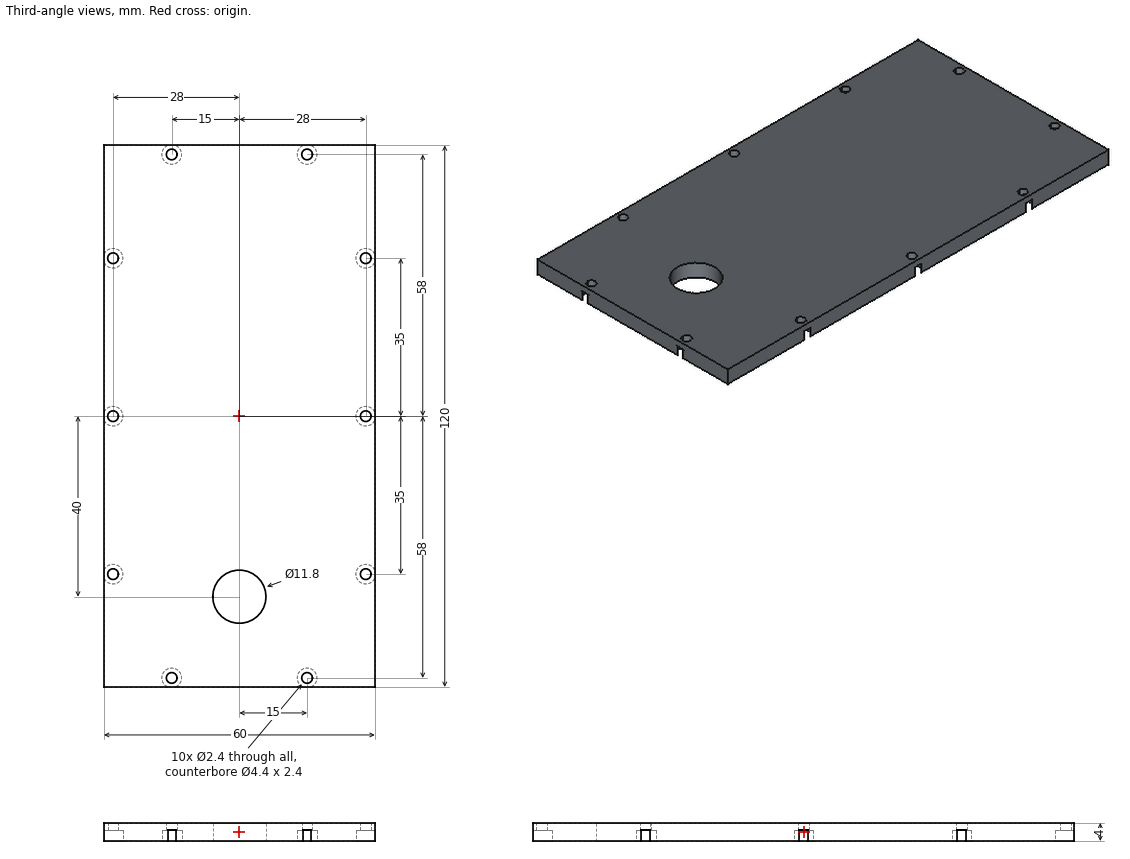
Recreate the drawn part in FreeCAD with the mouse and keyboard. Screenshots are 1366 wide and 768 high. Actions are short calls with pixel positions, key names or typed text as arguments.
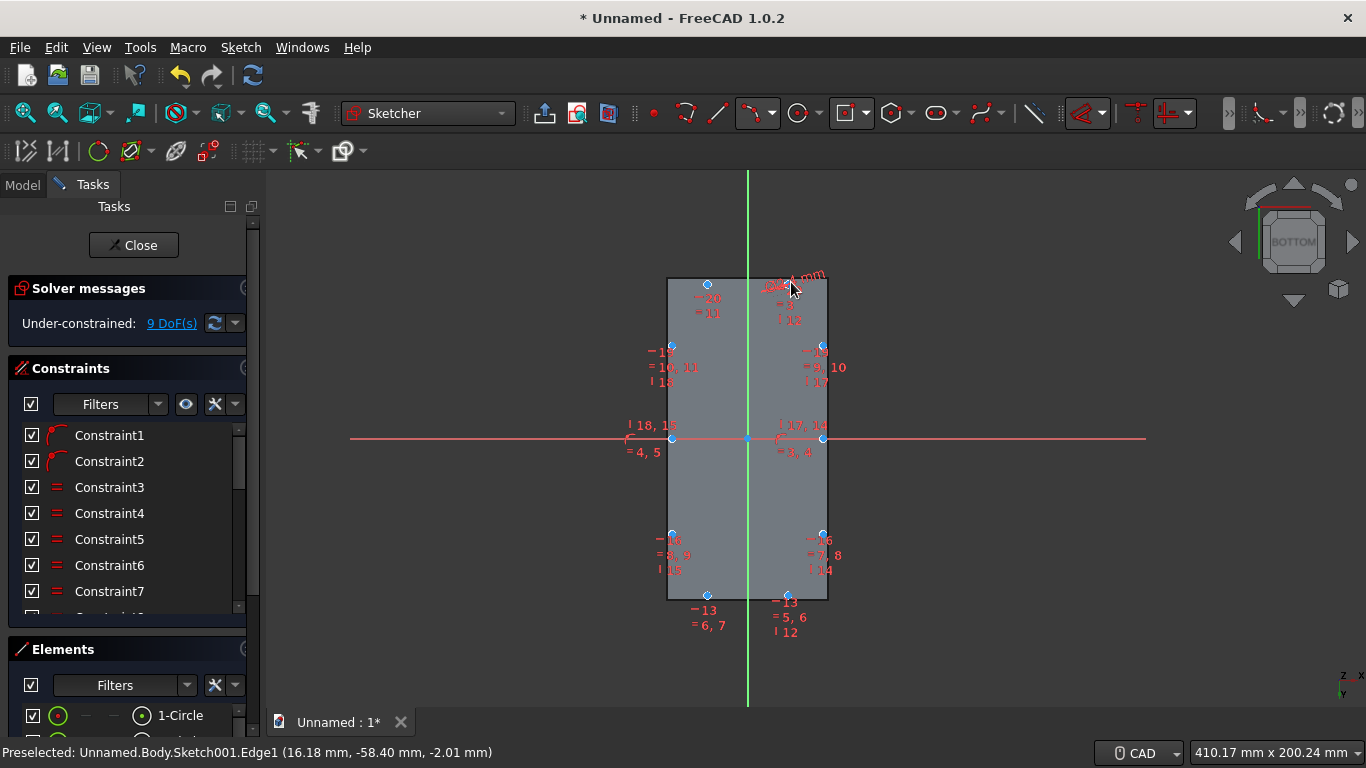
click(788, 284)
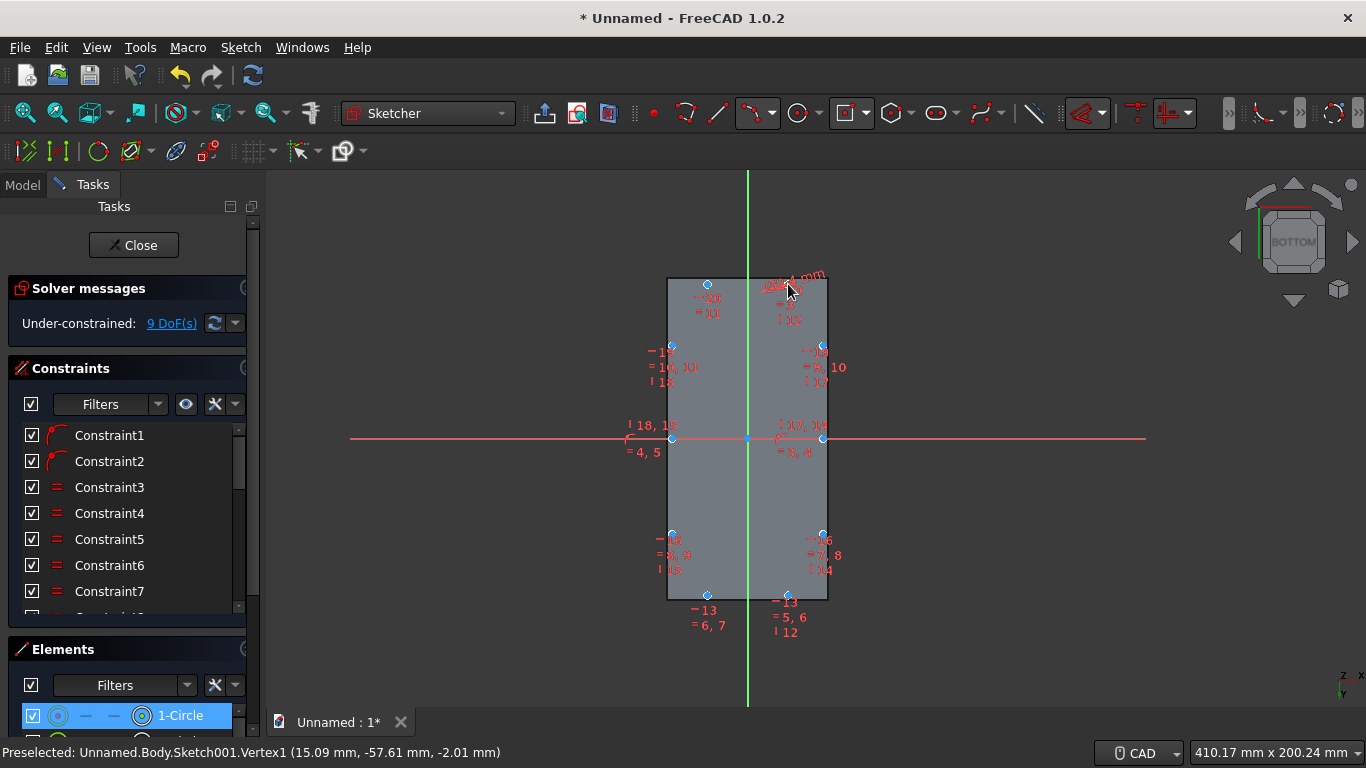
click(1104, 114)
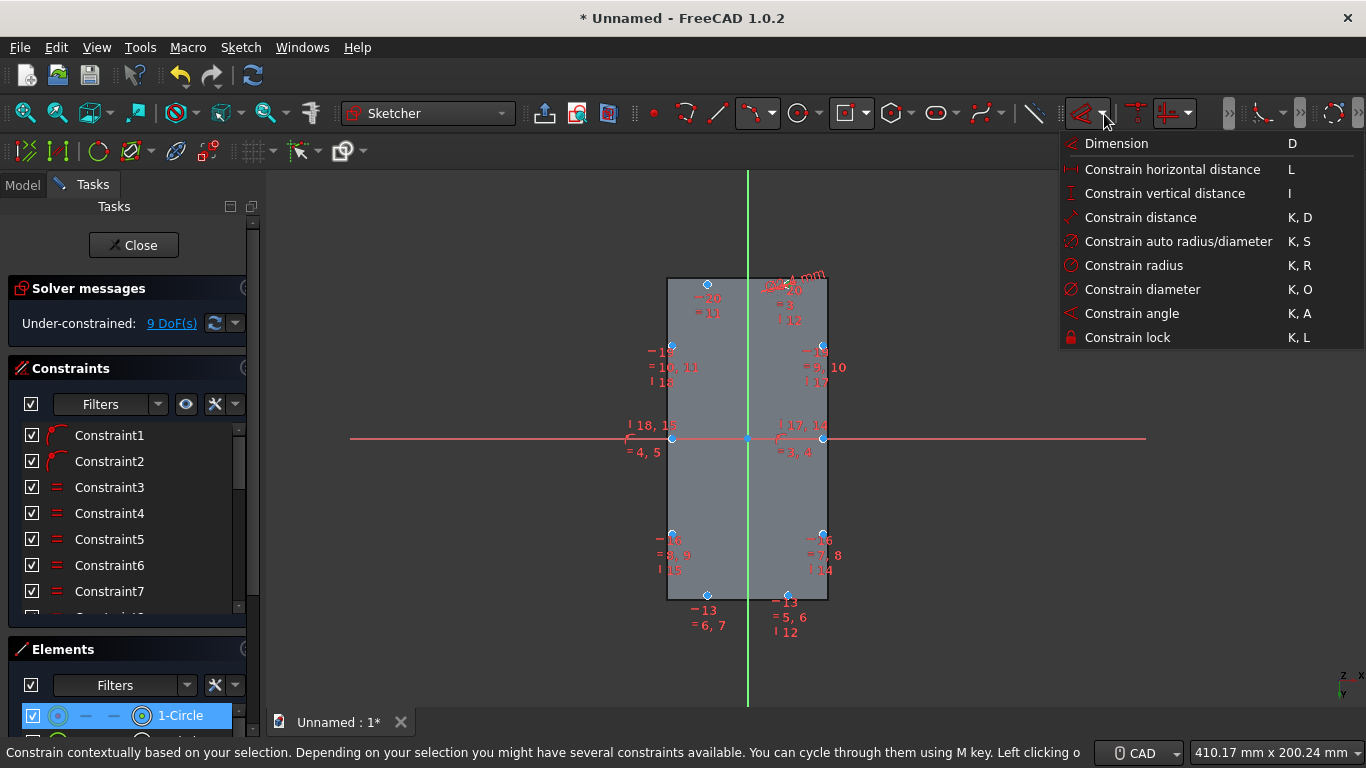
click(1212, 169)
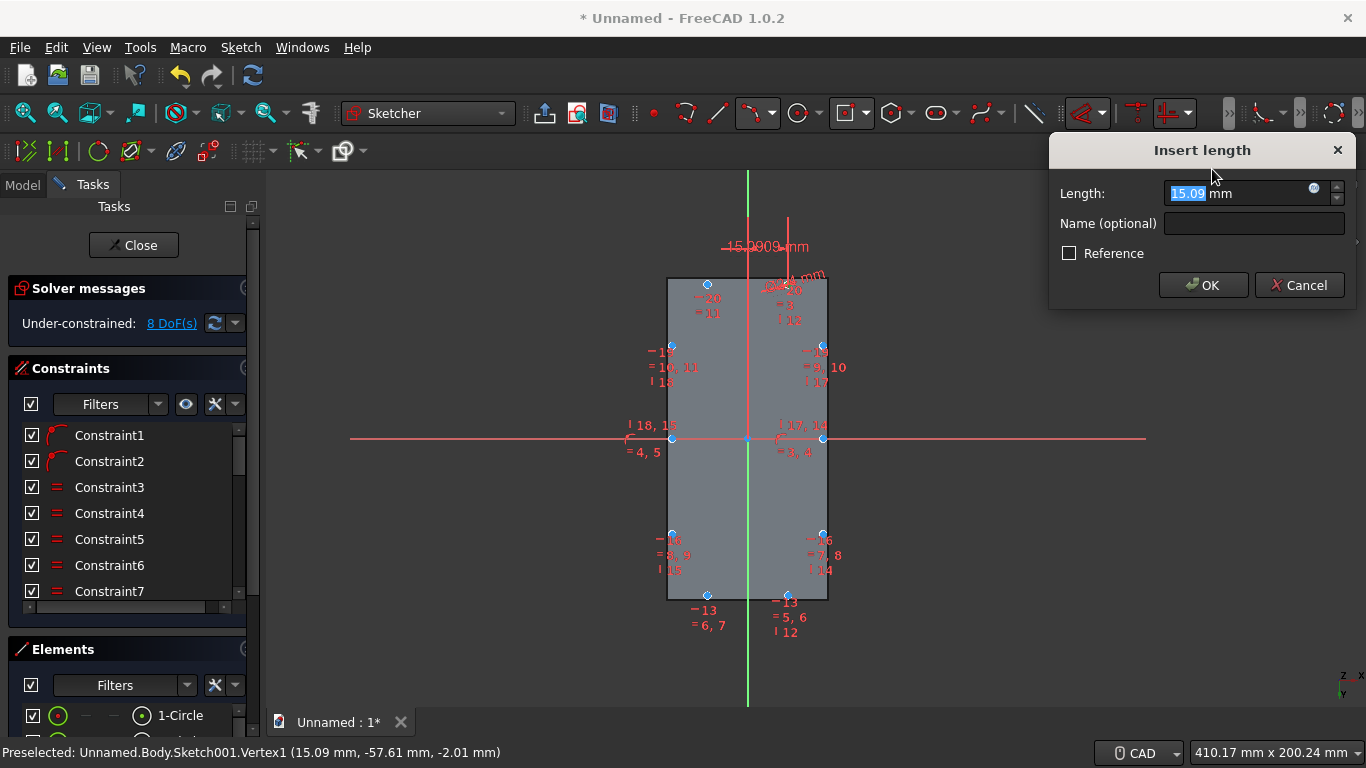
text(15)
key(Return)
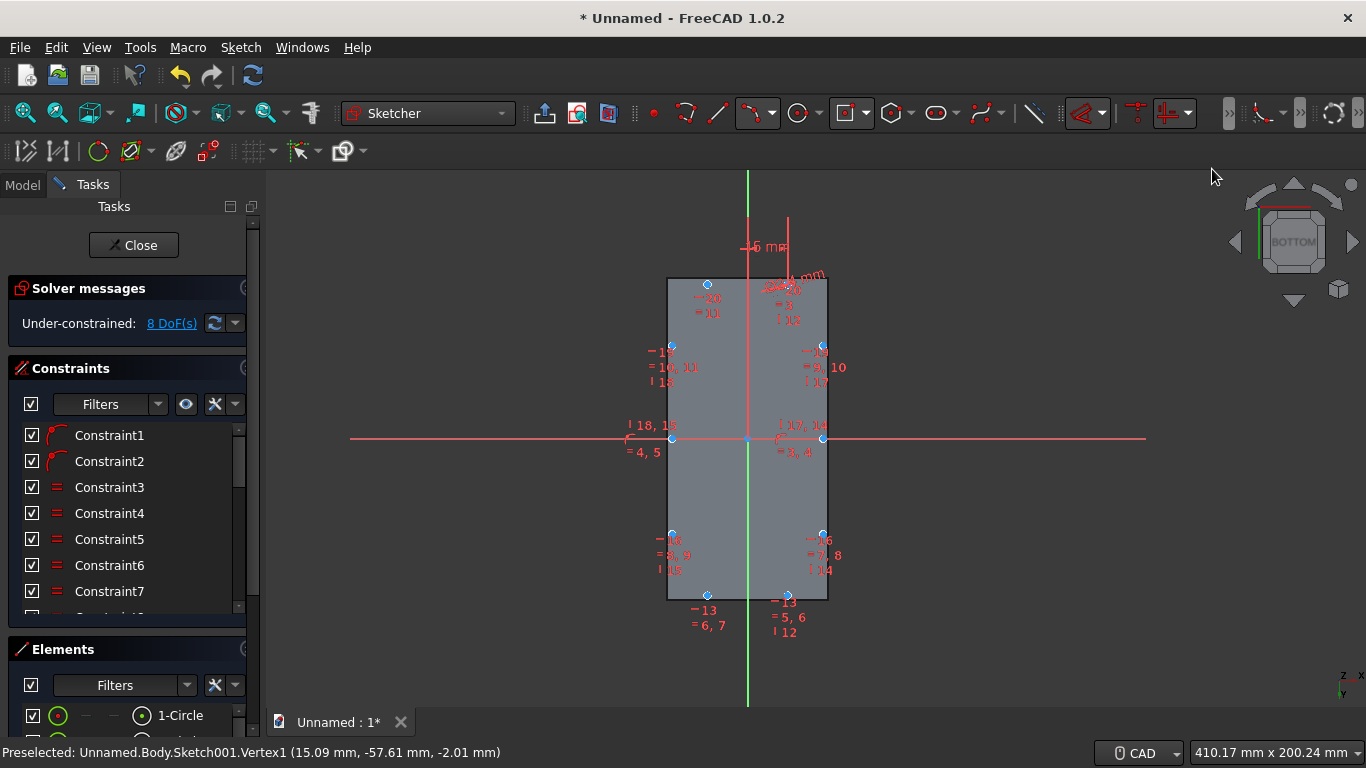
click(788, 284)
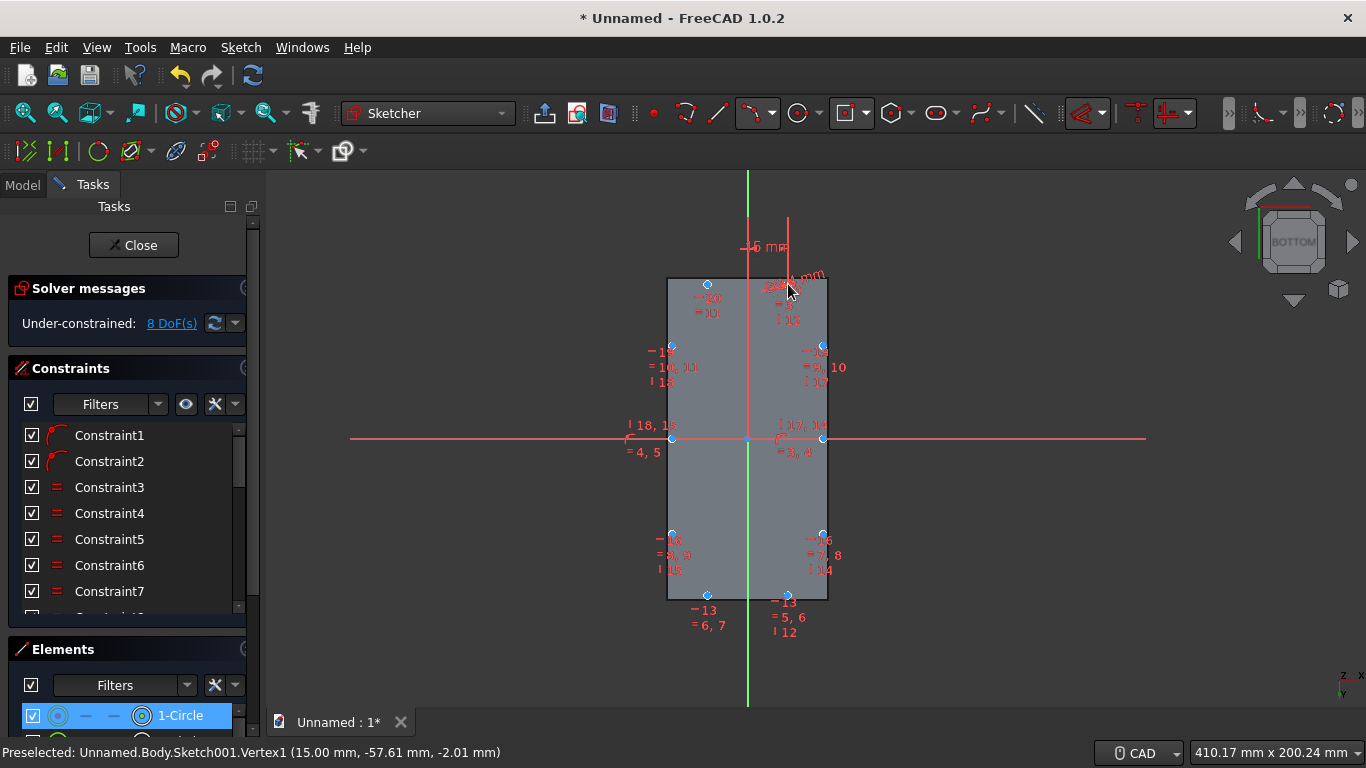
click(1104, 114)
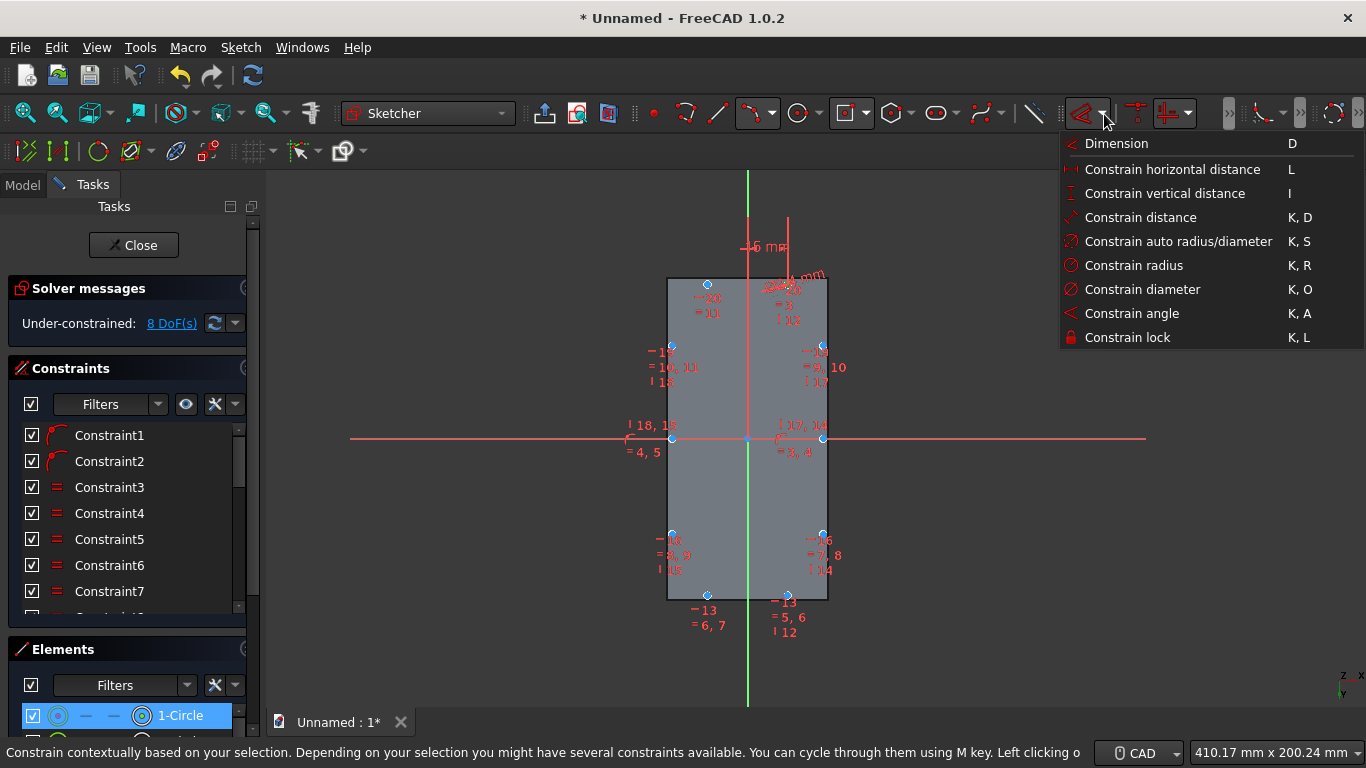
click(1212, 193)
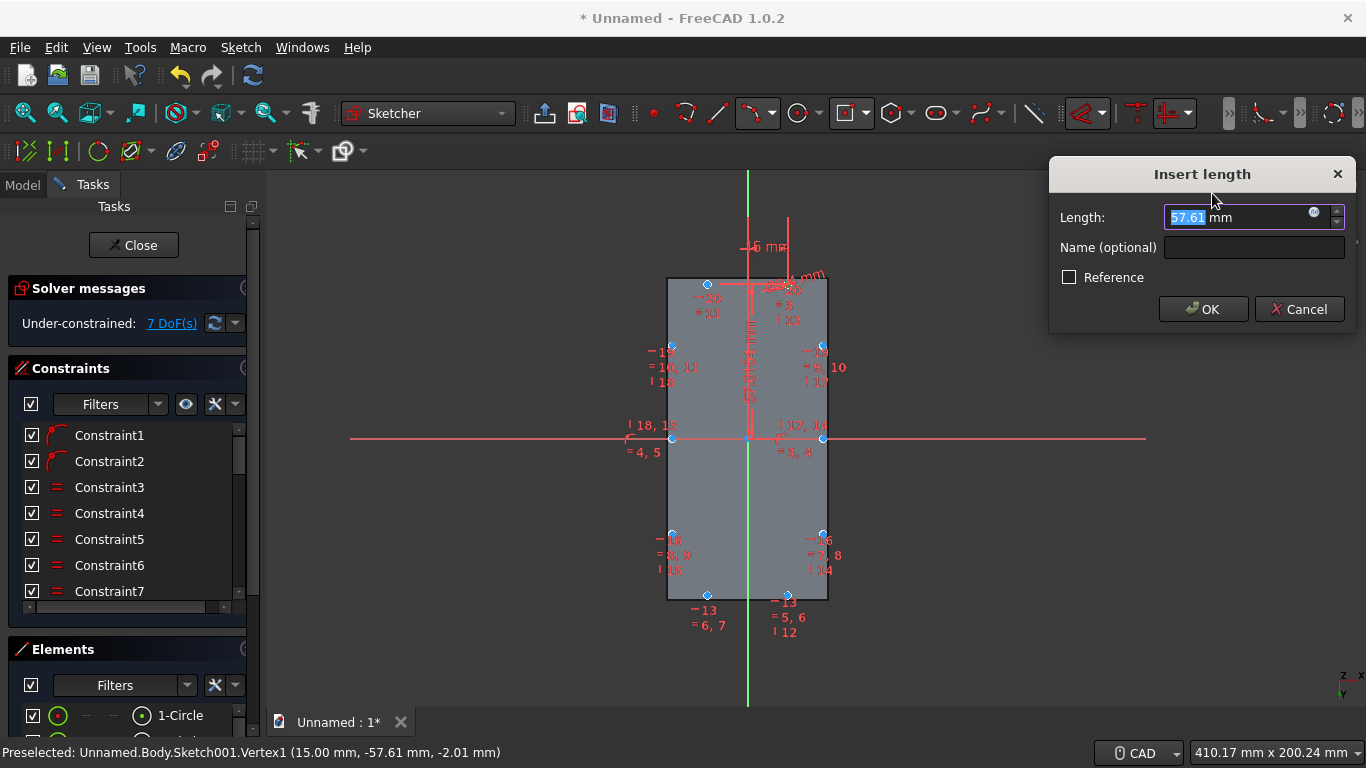
text(58)
key(Return)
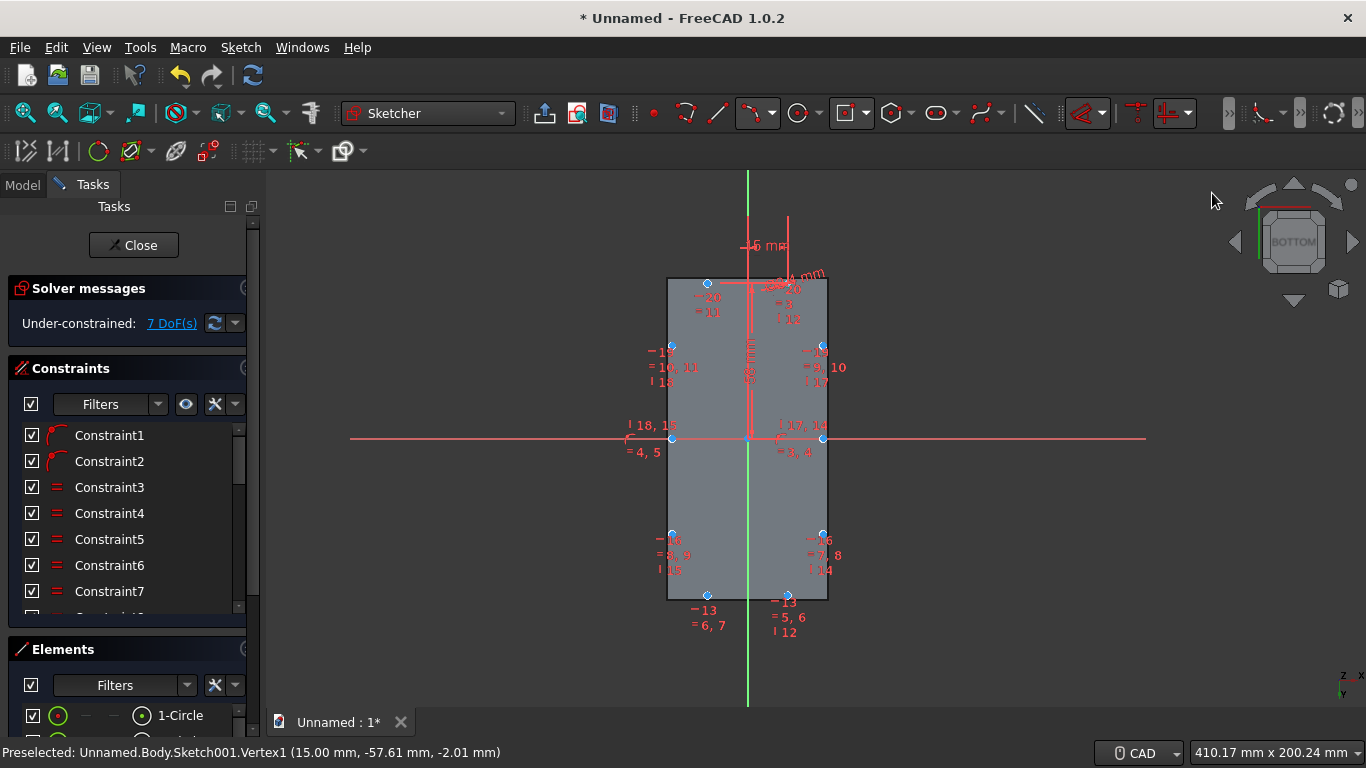
click(823, 439)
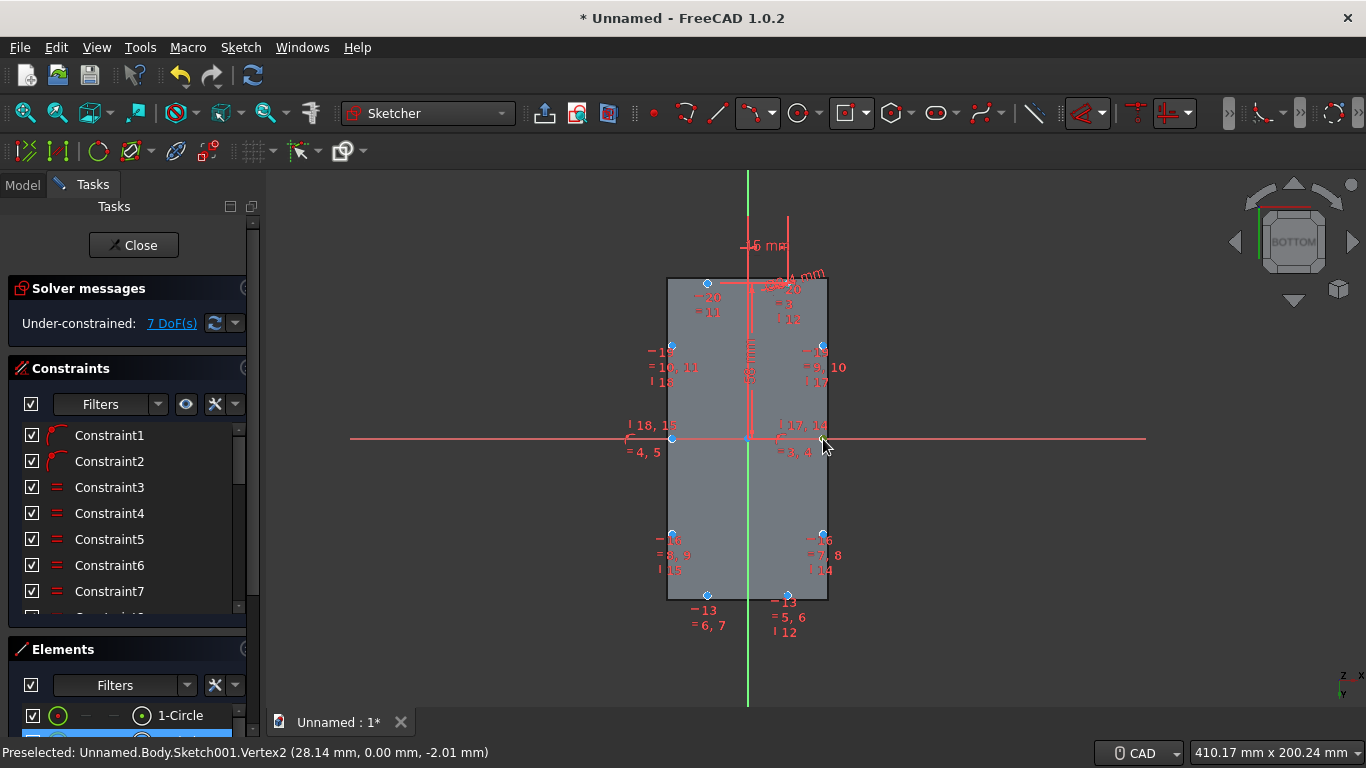
key(l)